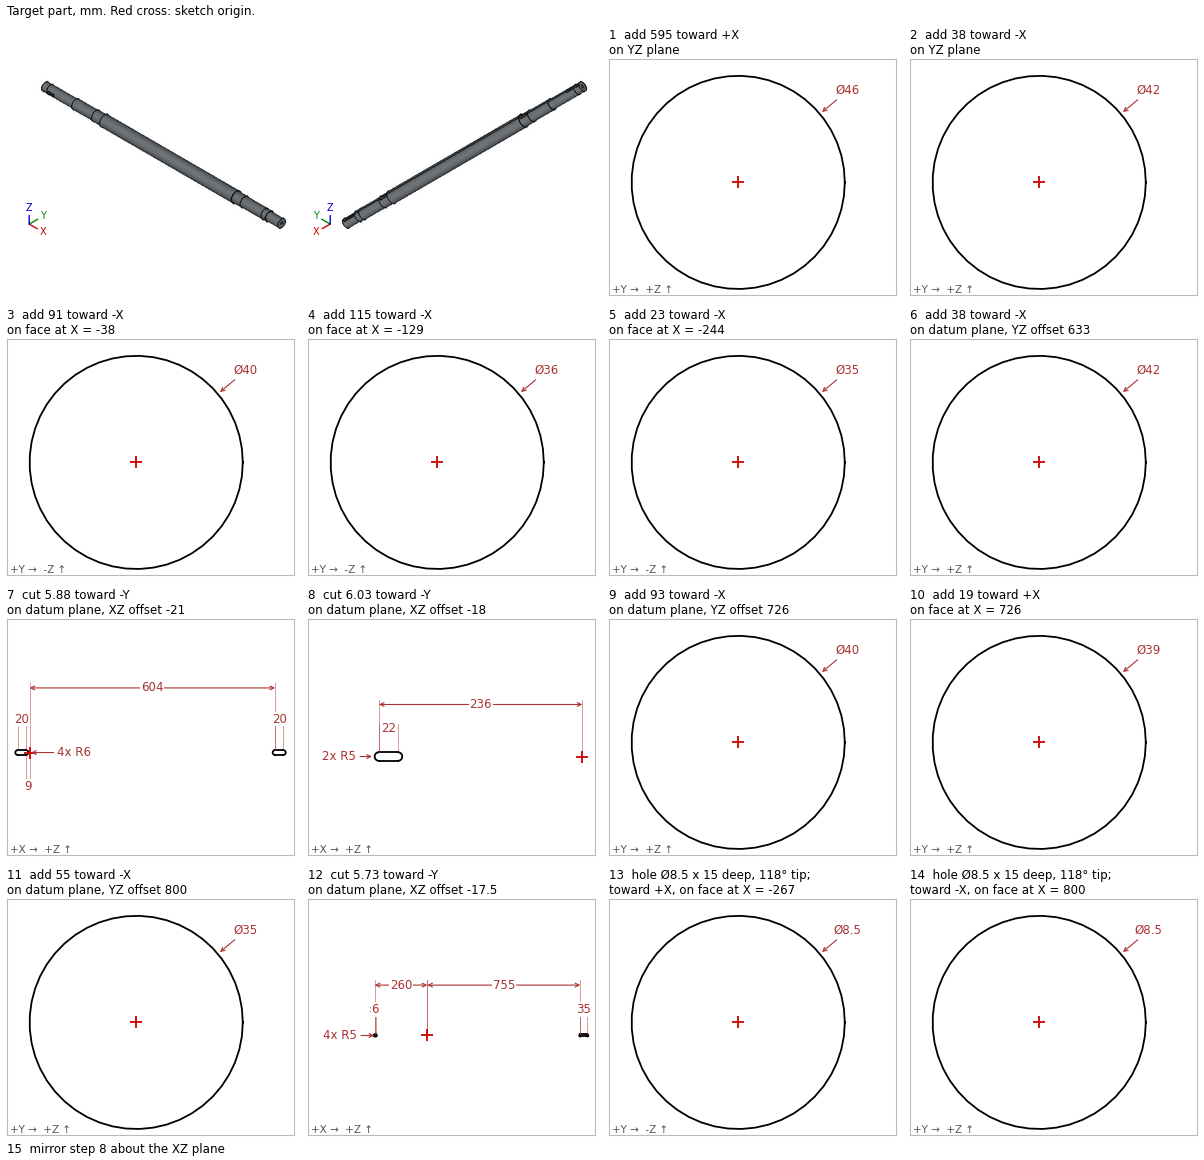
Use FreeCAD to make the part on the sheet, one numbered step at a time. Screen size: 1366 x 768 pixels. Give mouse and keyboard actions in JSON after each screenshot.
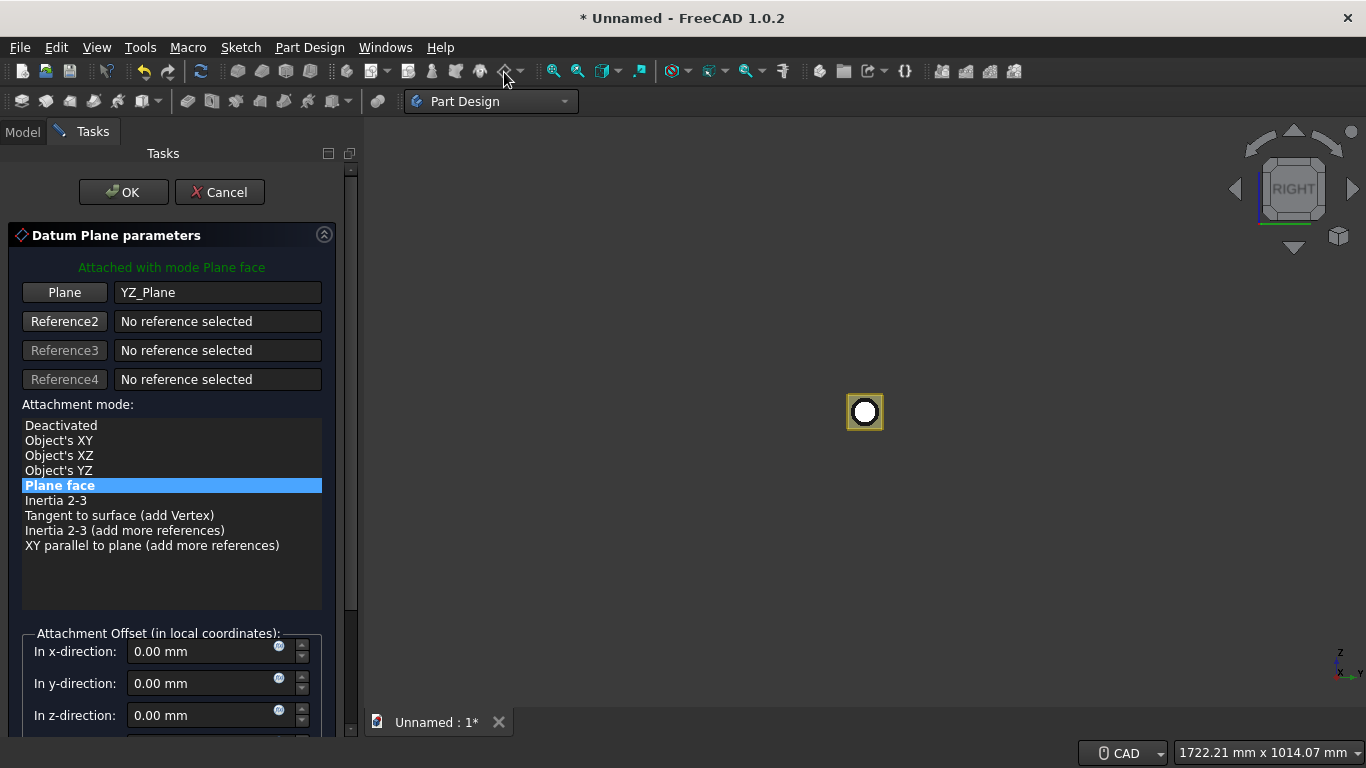
{"action": "triple_click", "coordinate": [210, 715]}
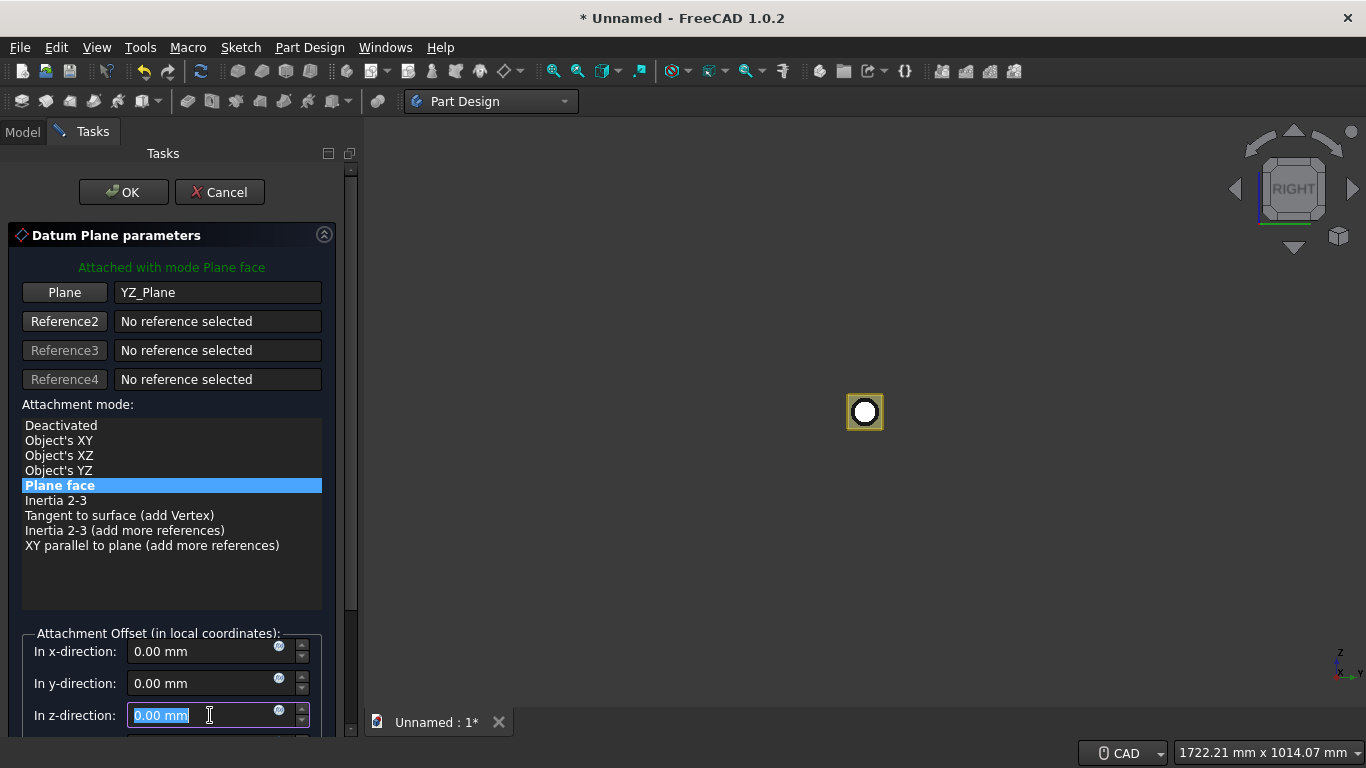
{"action": "type", "text": "800"}
{"action": "key", "text": "Tab"}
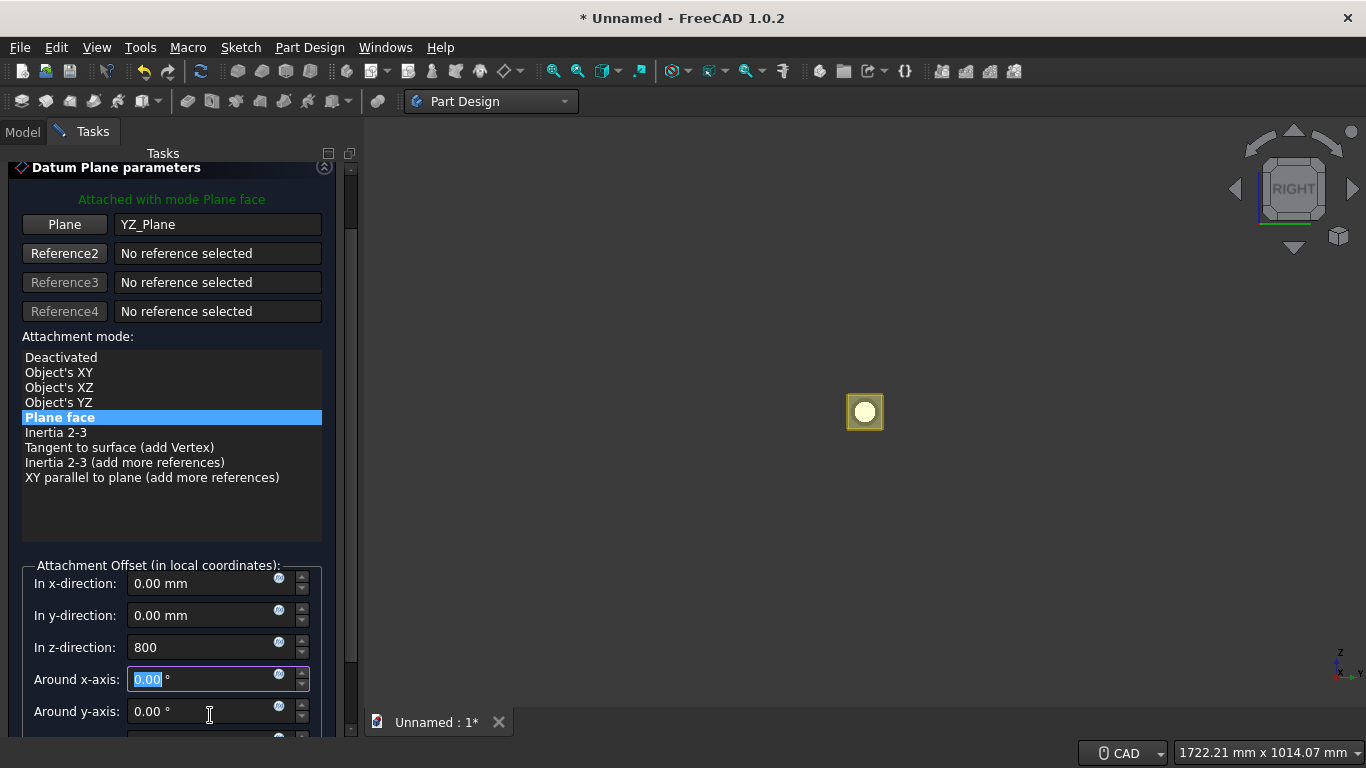
{"action": "scroll", "coordinate": [351, 450], "scroll_direction": "up", "scroll_amount": 2}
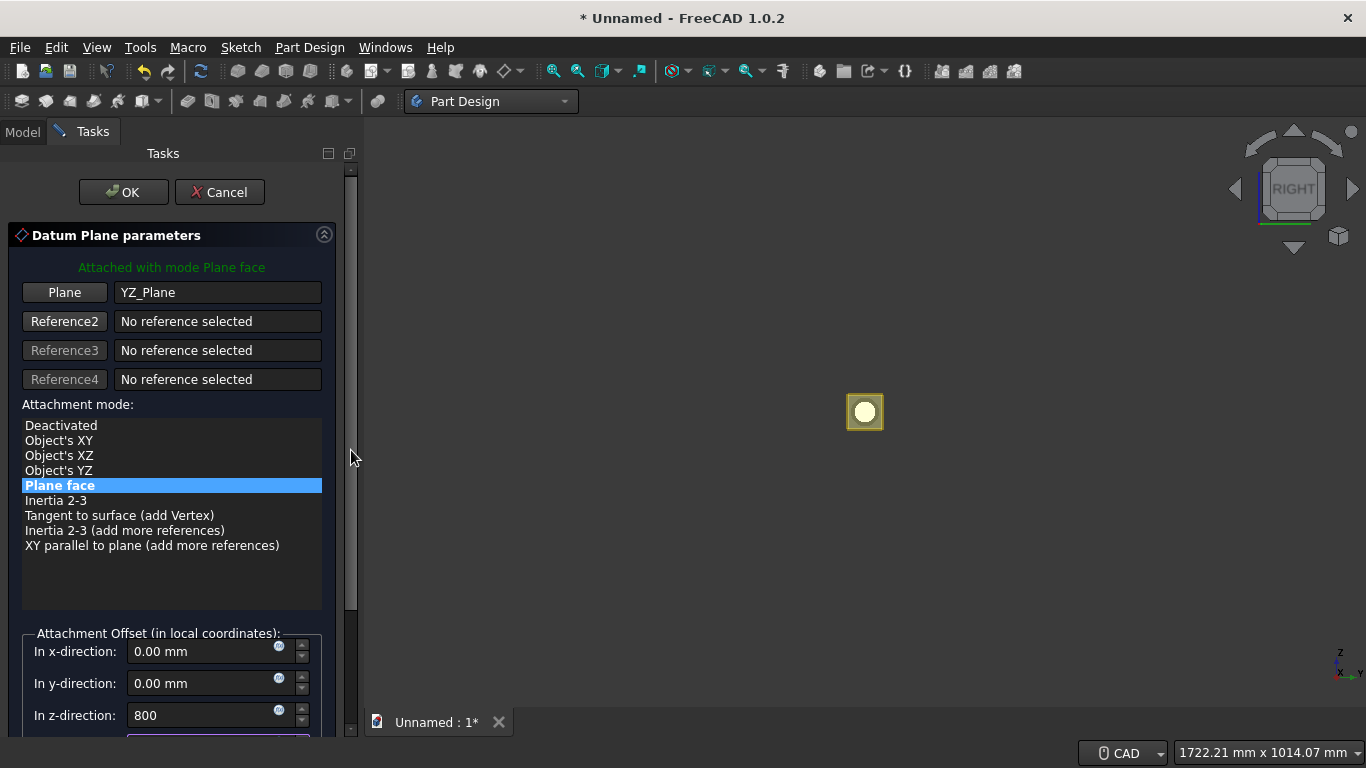
{"action": "left_click", "coordinate": [124, 192]}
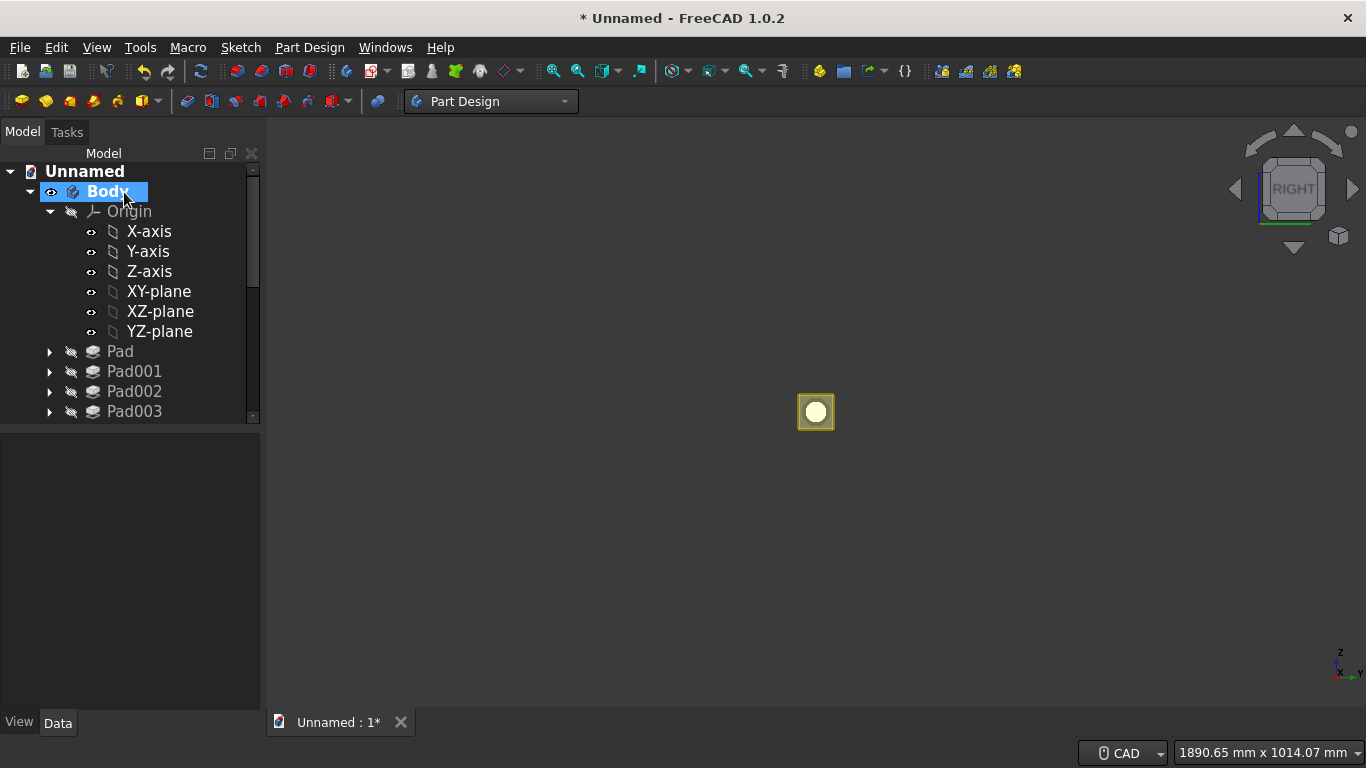
{"action": "scroll", "coordinate": [100, 287], "scroll_direction": "down", "scroll_amount": 3}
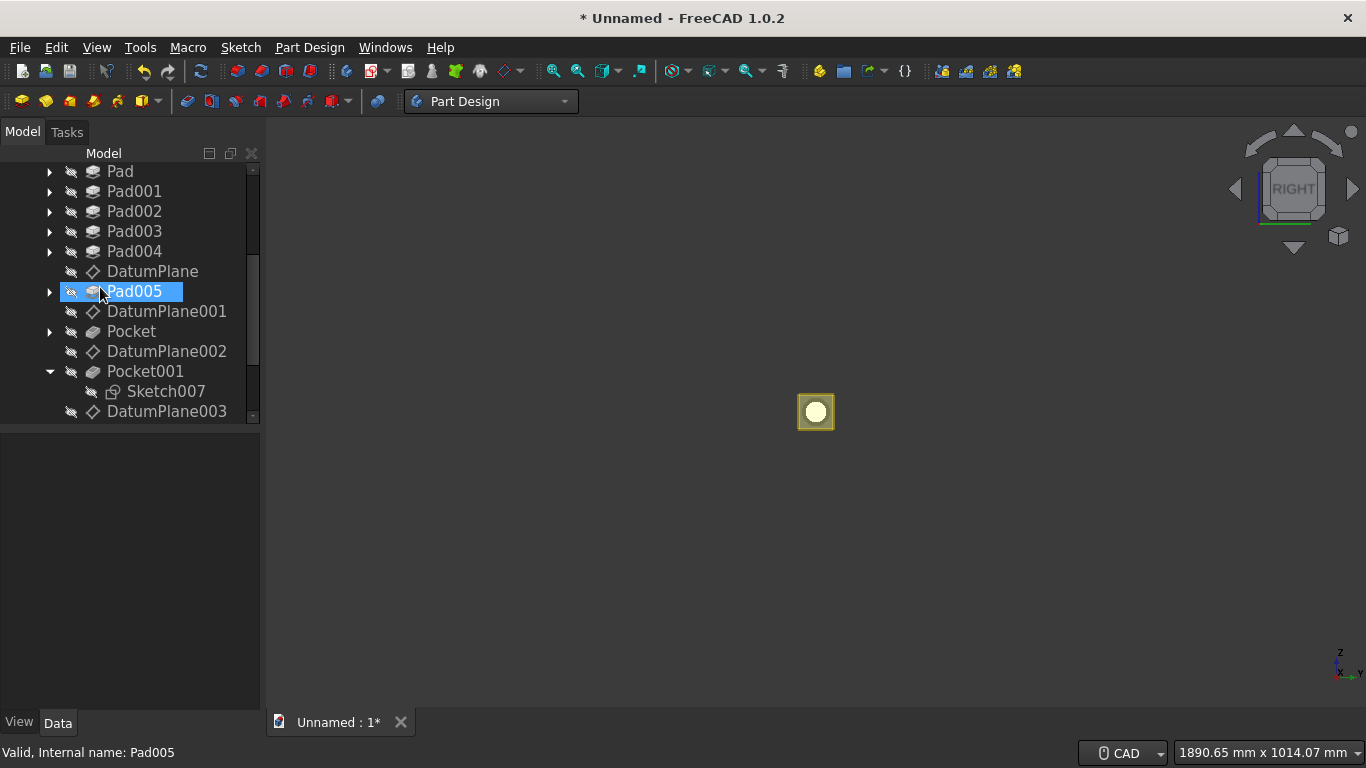
{"action": "scroll", "coordinate": [140, 287], "scroll_direction": "up", "scroll_amount": 15}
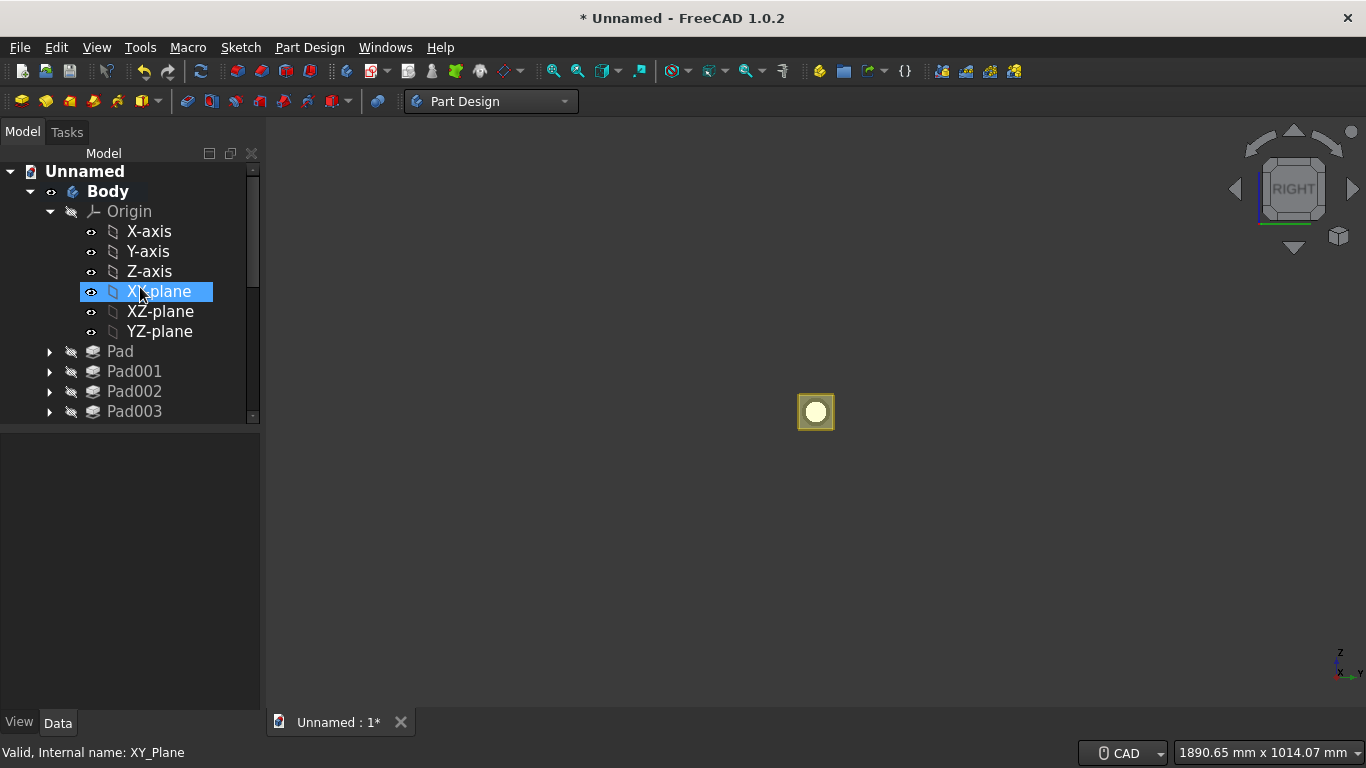
{"action": "scroll", "coordinate": [100, 287], "scroll_direction": "down", "scroll_amount": 6}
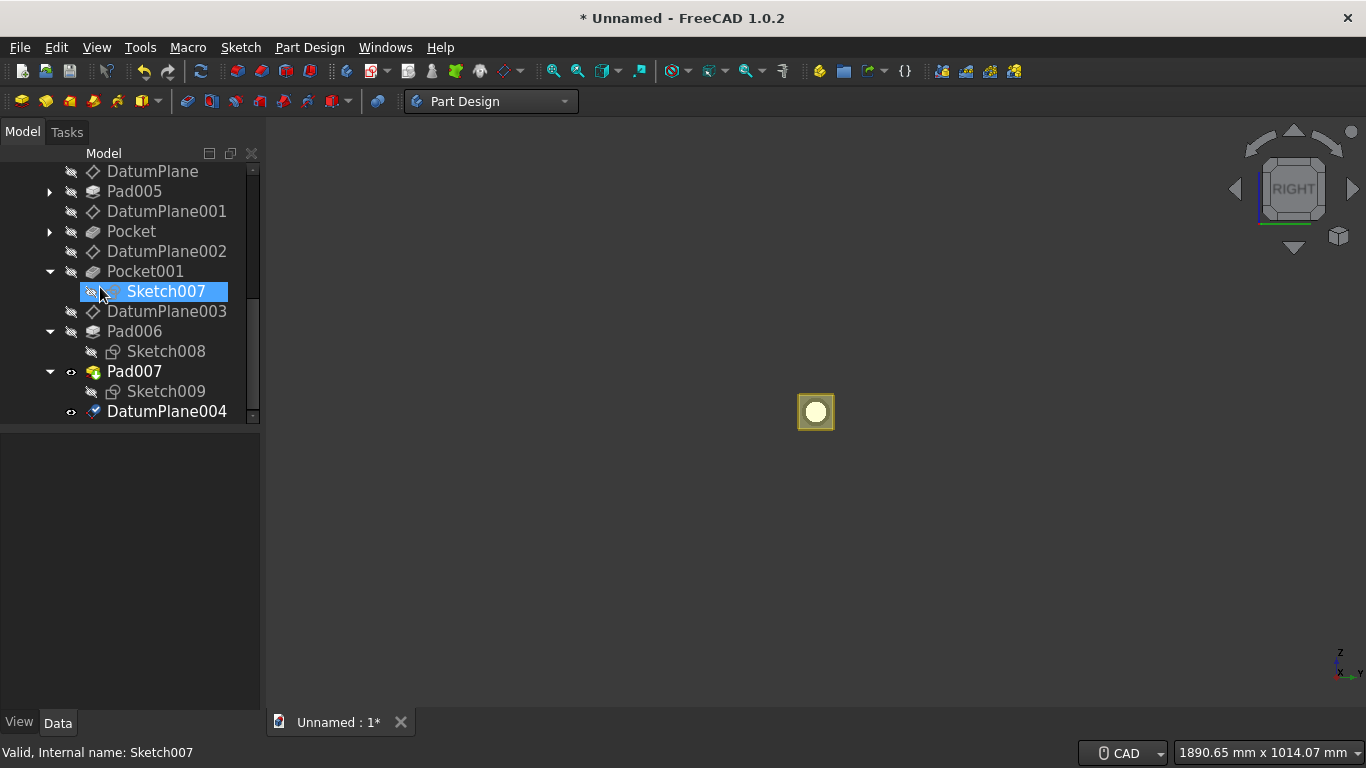
{"action": "left_click", "coordinate": [116, 412]}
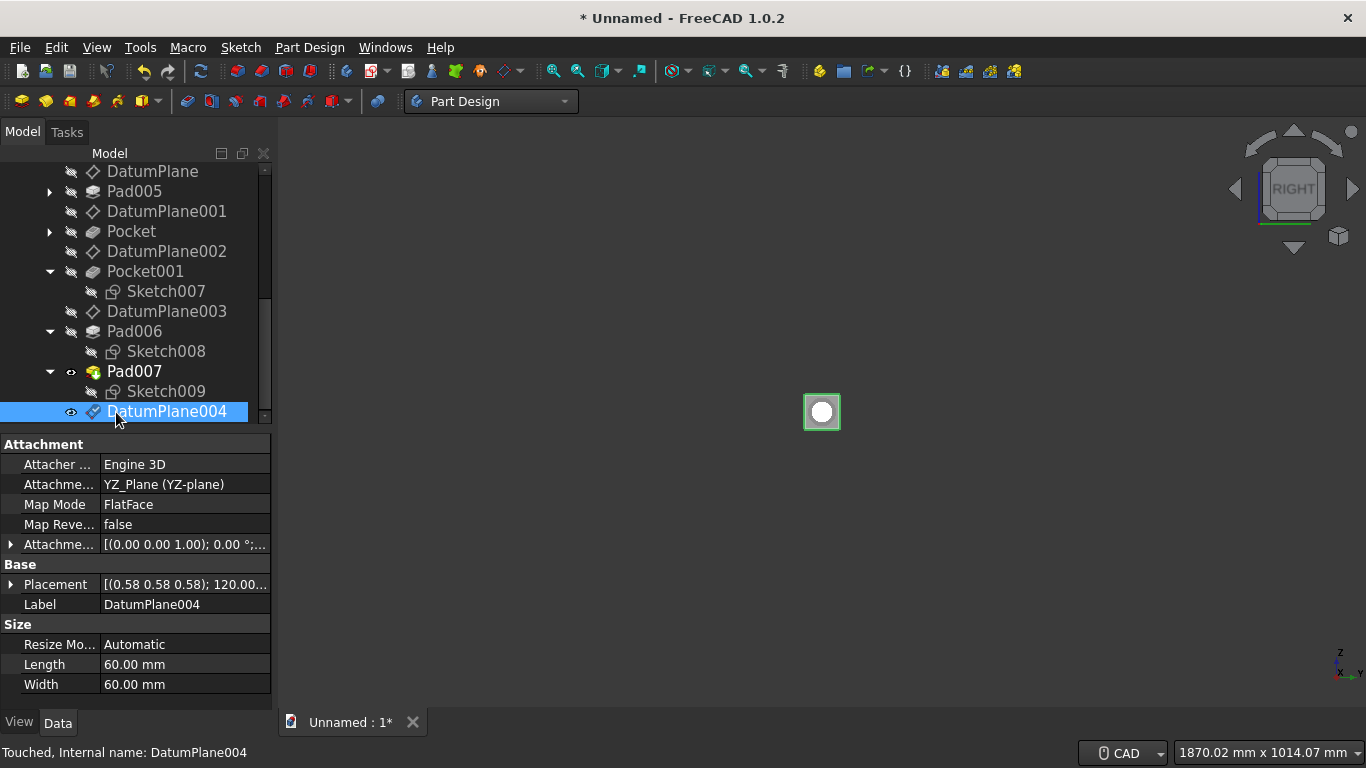
{"action": "left_click", "coordinate": [372, 72]}